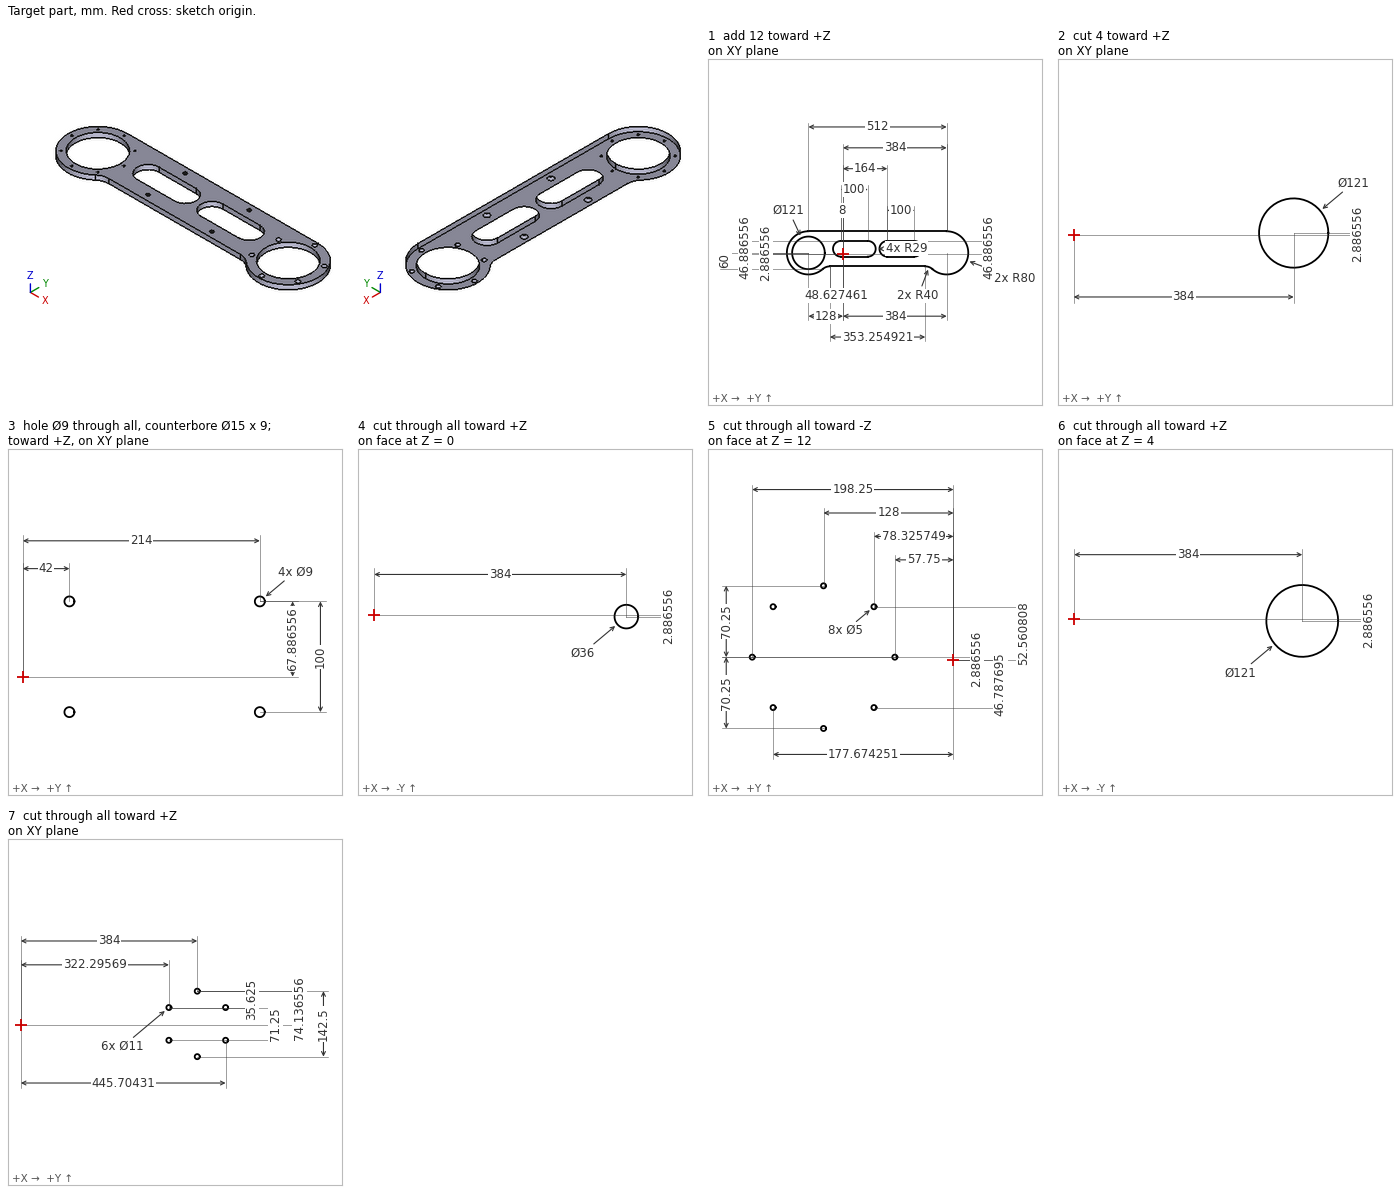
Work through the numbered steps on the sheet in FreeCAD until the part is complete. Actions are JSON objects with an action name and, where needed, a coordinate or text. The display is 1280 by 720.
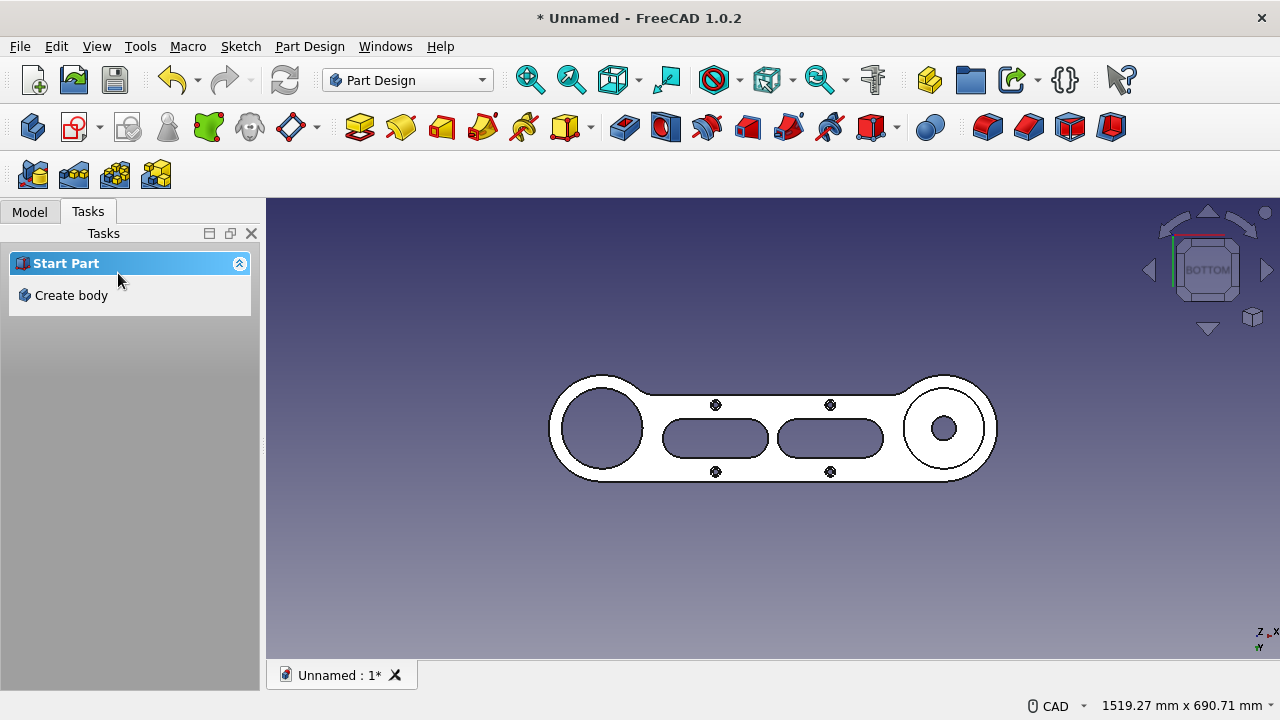
{"action": "left_click", "coordinate": [531, 80]}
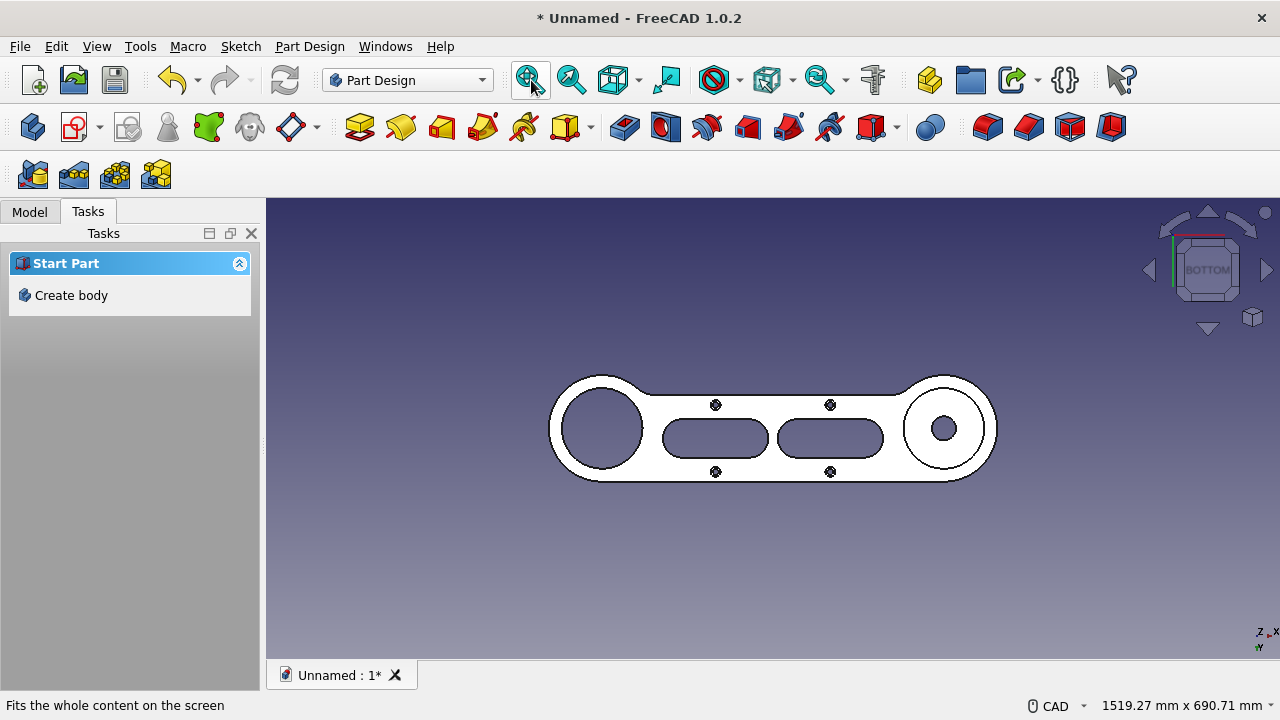
{"action": "key", "text": "0"}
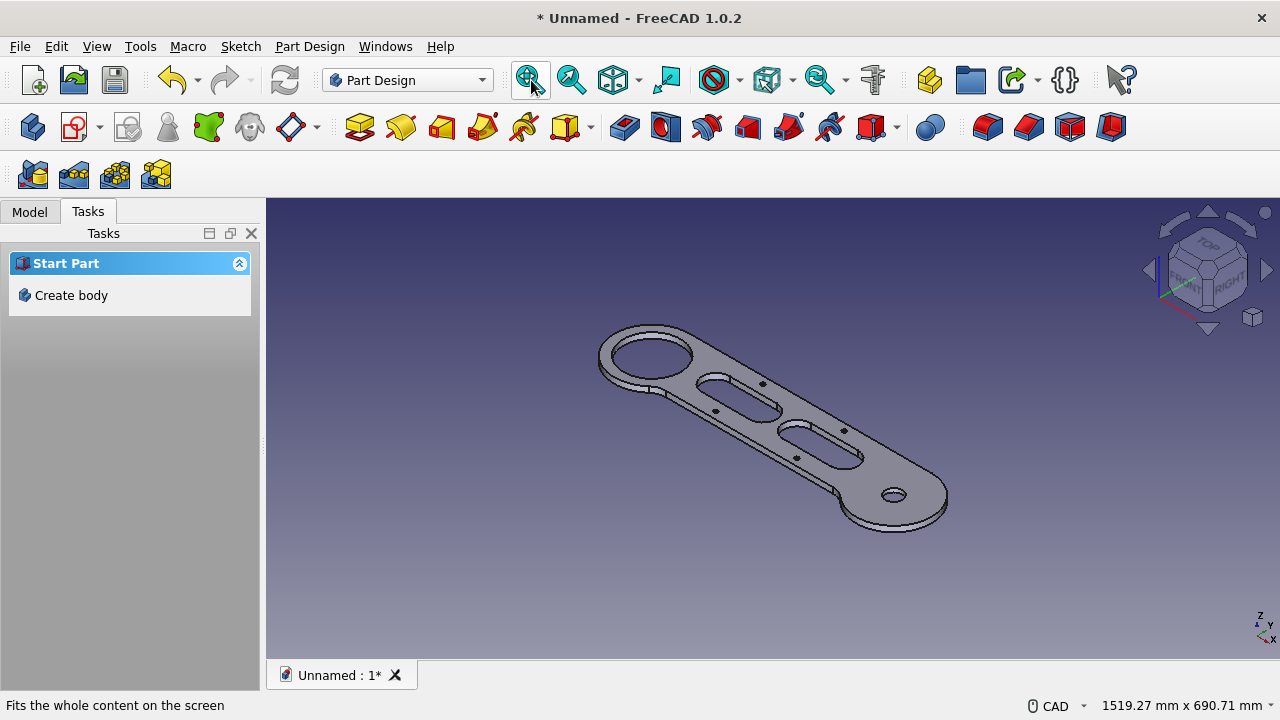
{"action": "left_click", "coordinate": [885, 464]}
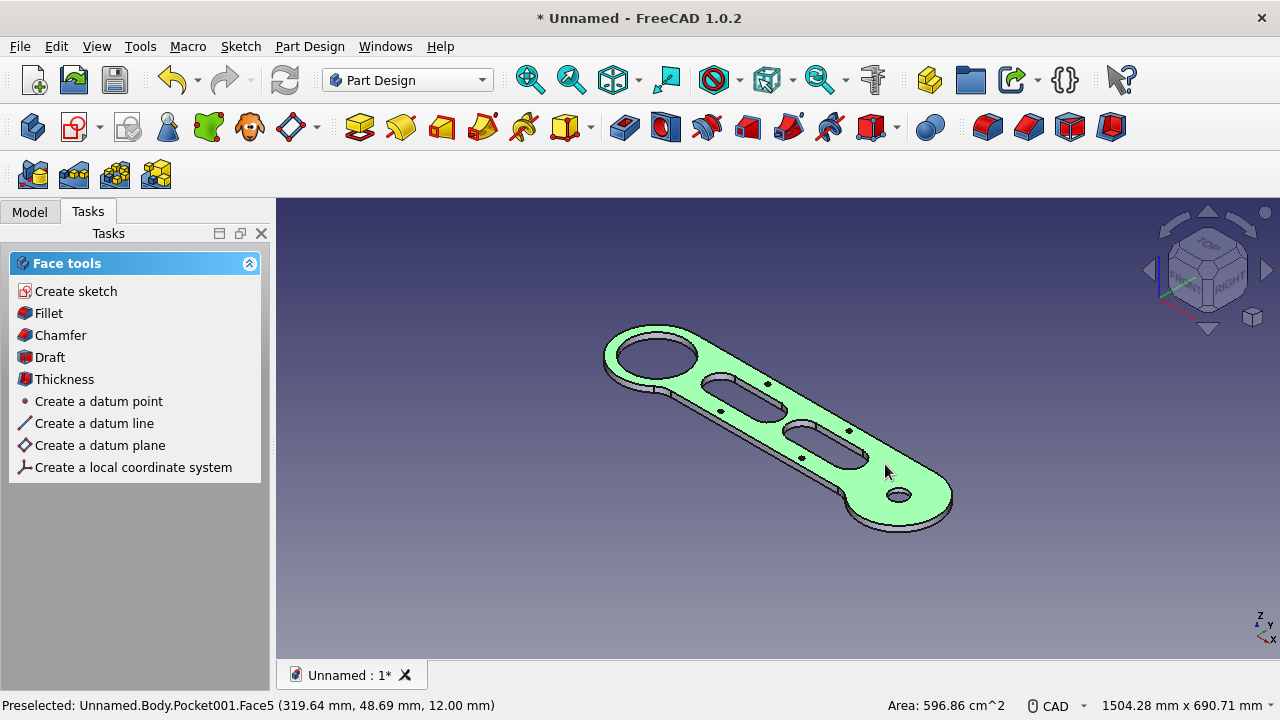
{"action": "left_click", "coordinate": [74, 128]}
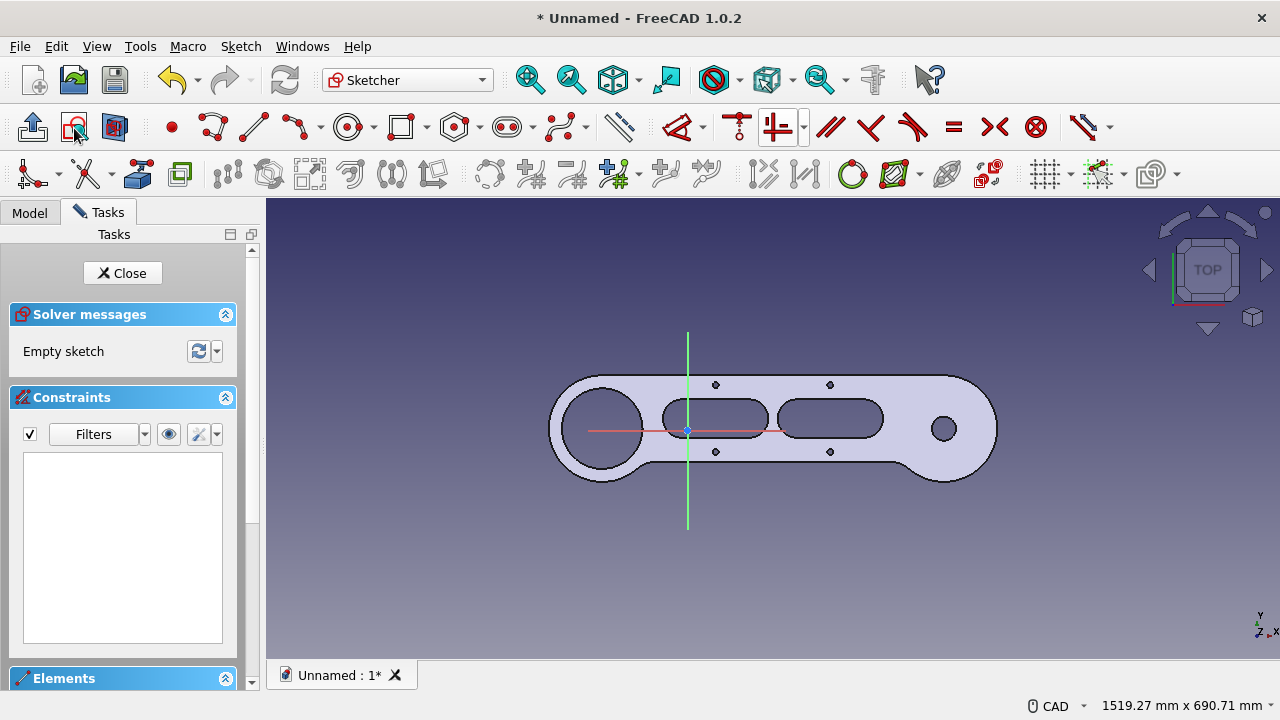
{"action": "scroll", "coordinate": [572, 429], "scroll_direction": "up", "scroll_amount": 5}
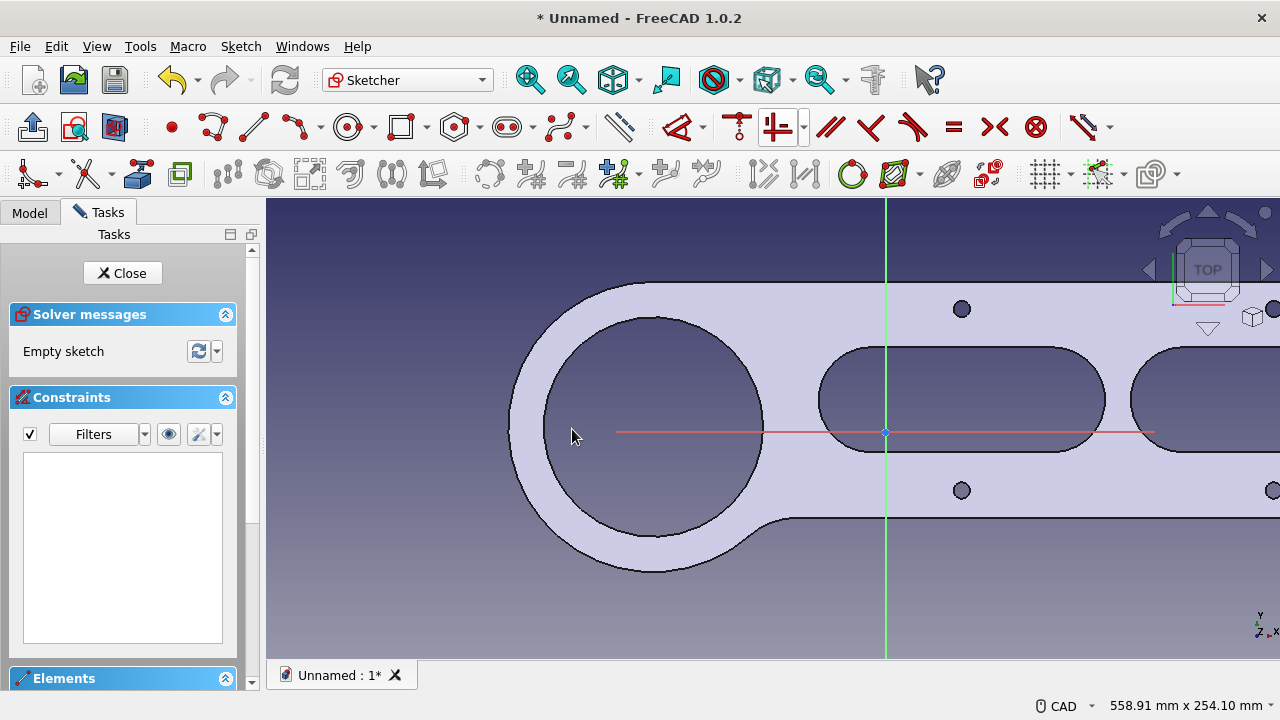
{"action": "left_click", "coordinate": [348, 128]}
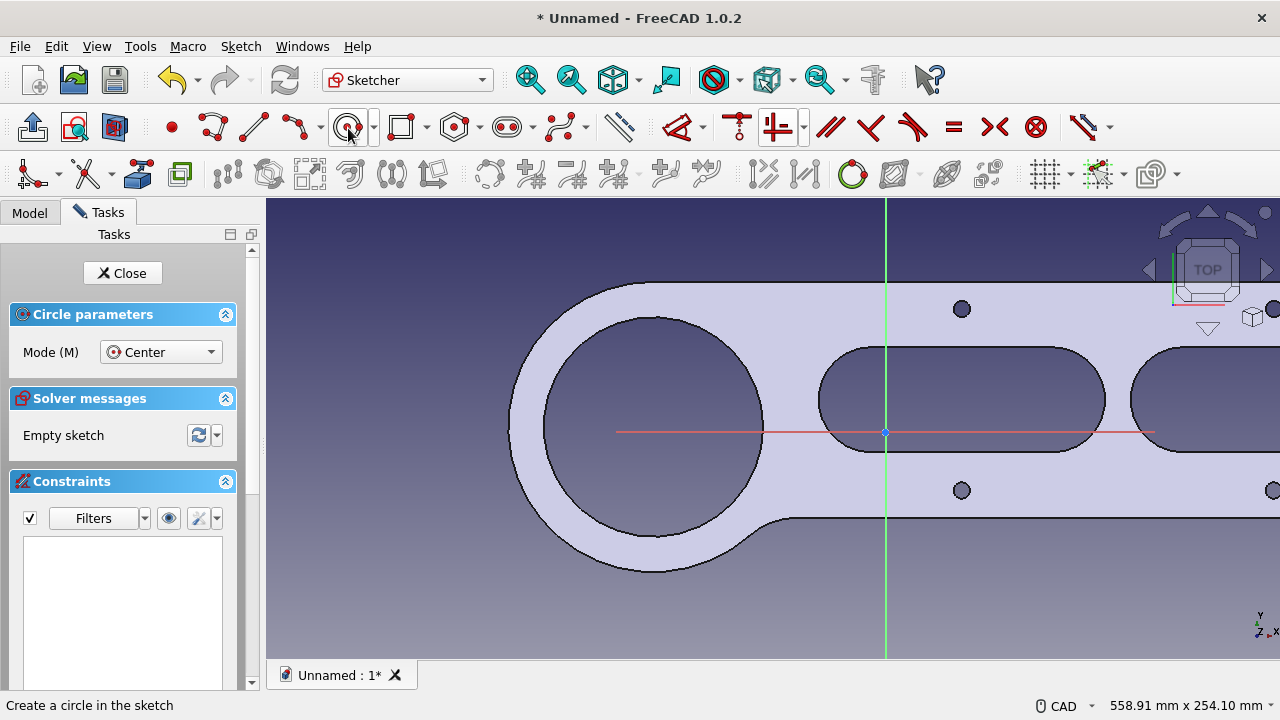
{"action": "scroll", "coordinate": [744, 337], "scroll_direction": "up", "scroll_amount": 9}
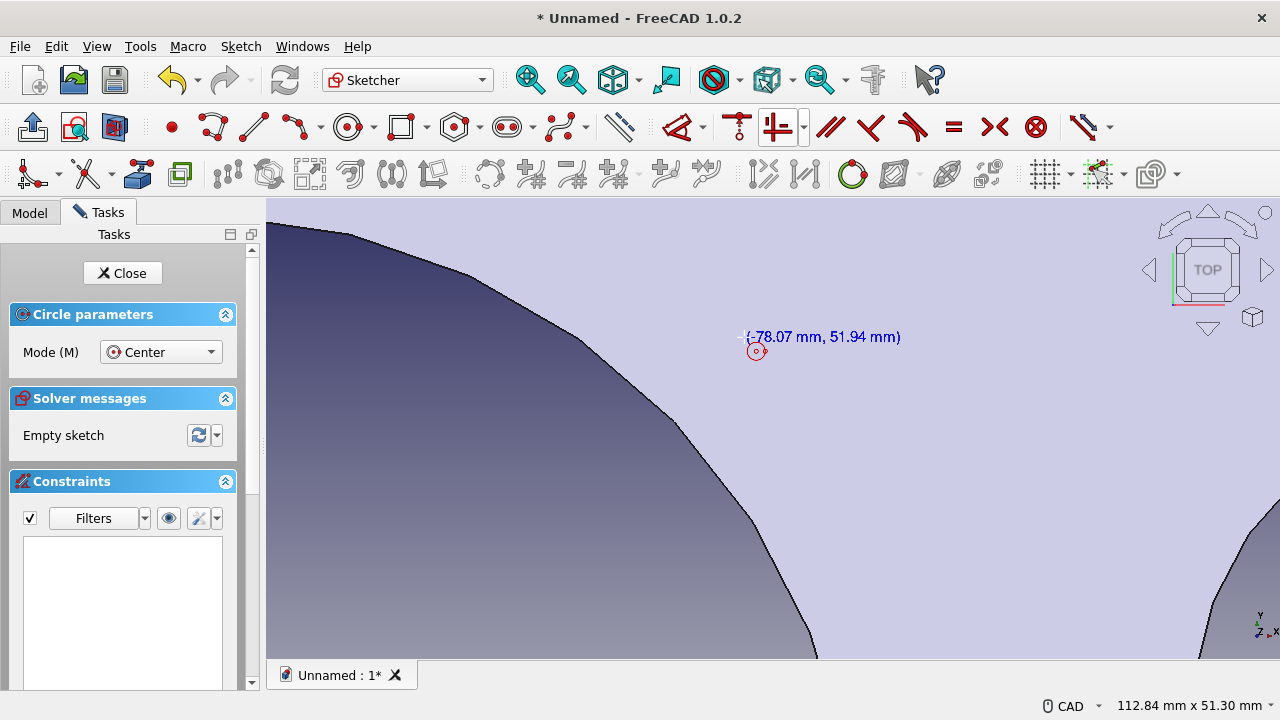
{"action": "scroll", "coordinate": [746, 339], "scroll_direction": "down", "scroll_amount": 9}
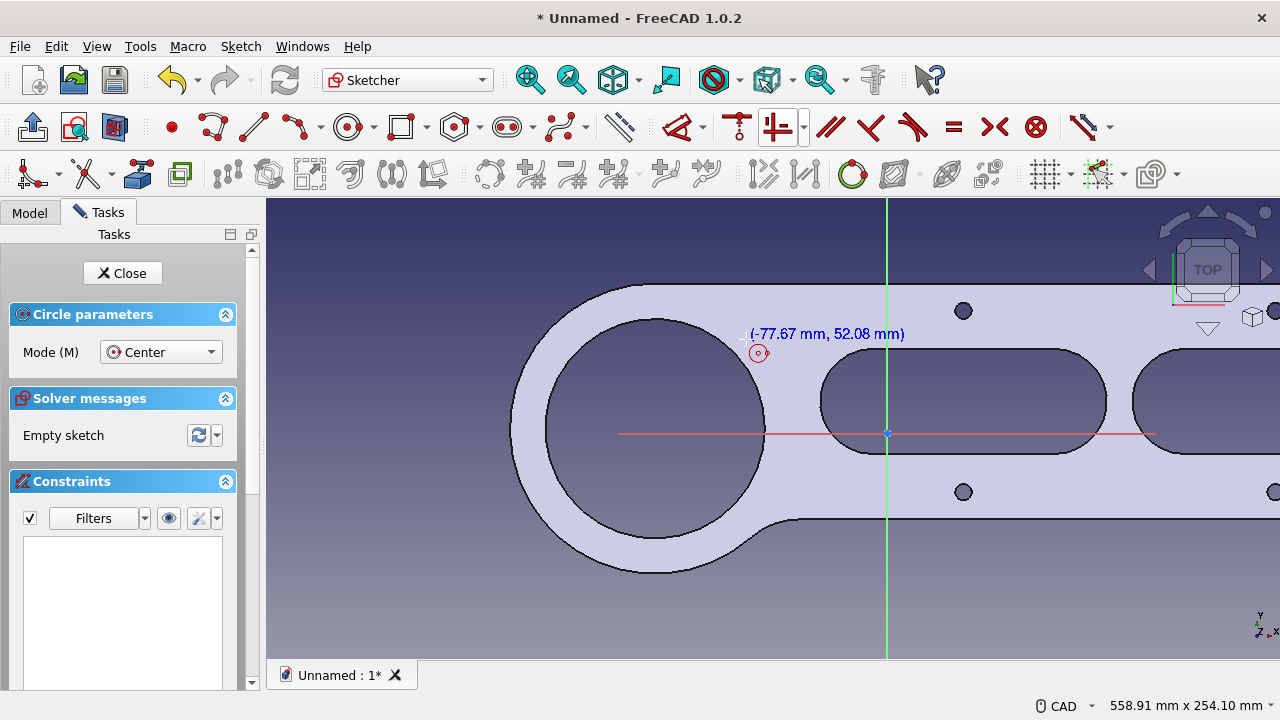
{"action": "left_click", "coordinate": [745, 339]}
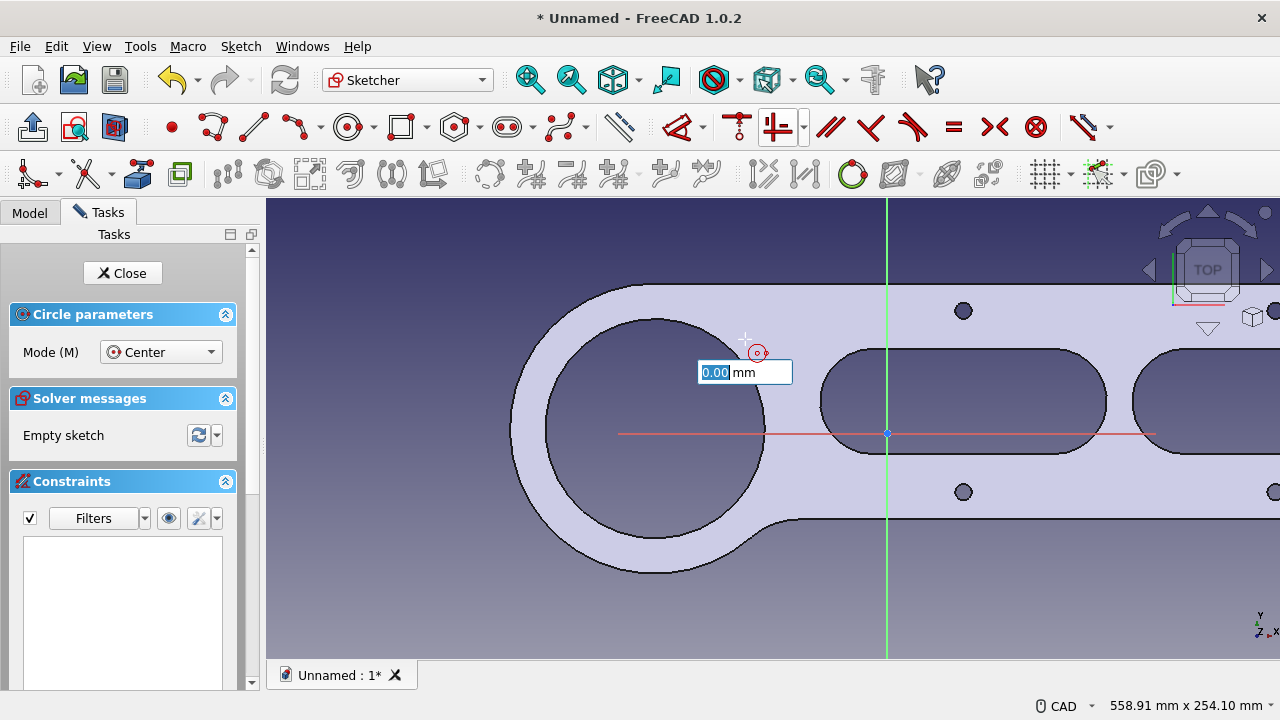
{"action": "scroll", "coordinate": [748, 335], "scroll_direction": "up", "scroll_amount": 7}